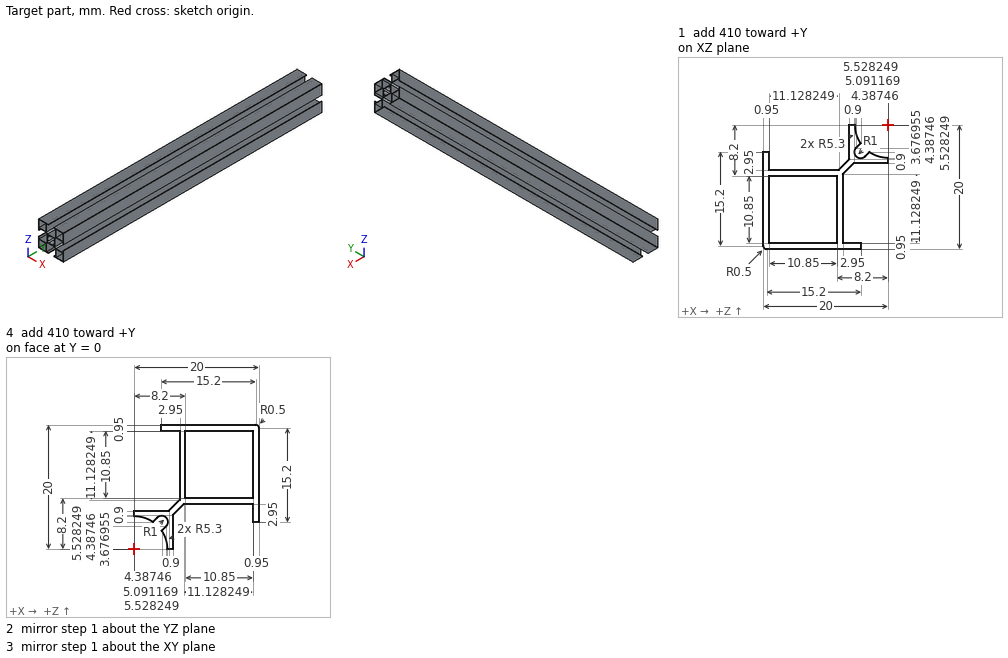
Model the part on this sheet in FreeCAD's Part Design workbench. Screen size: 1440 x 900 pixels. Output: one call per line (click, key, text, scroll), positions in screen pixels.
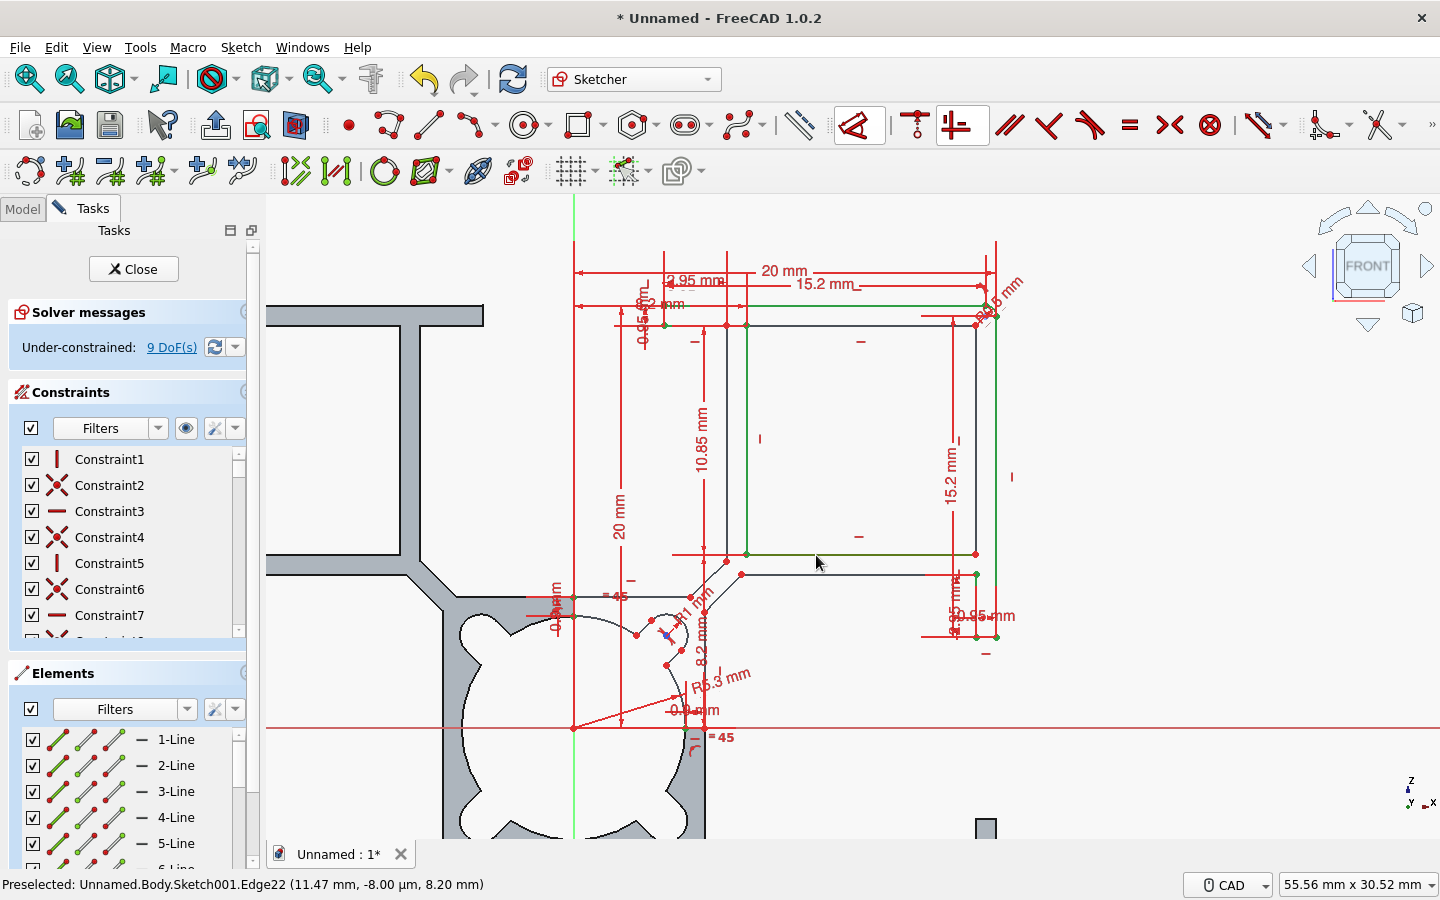
click(880, 126)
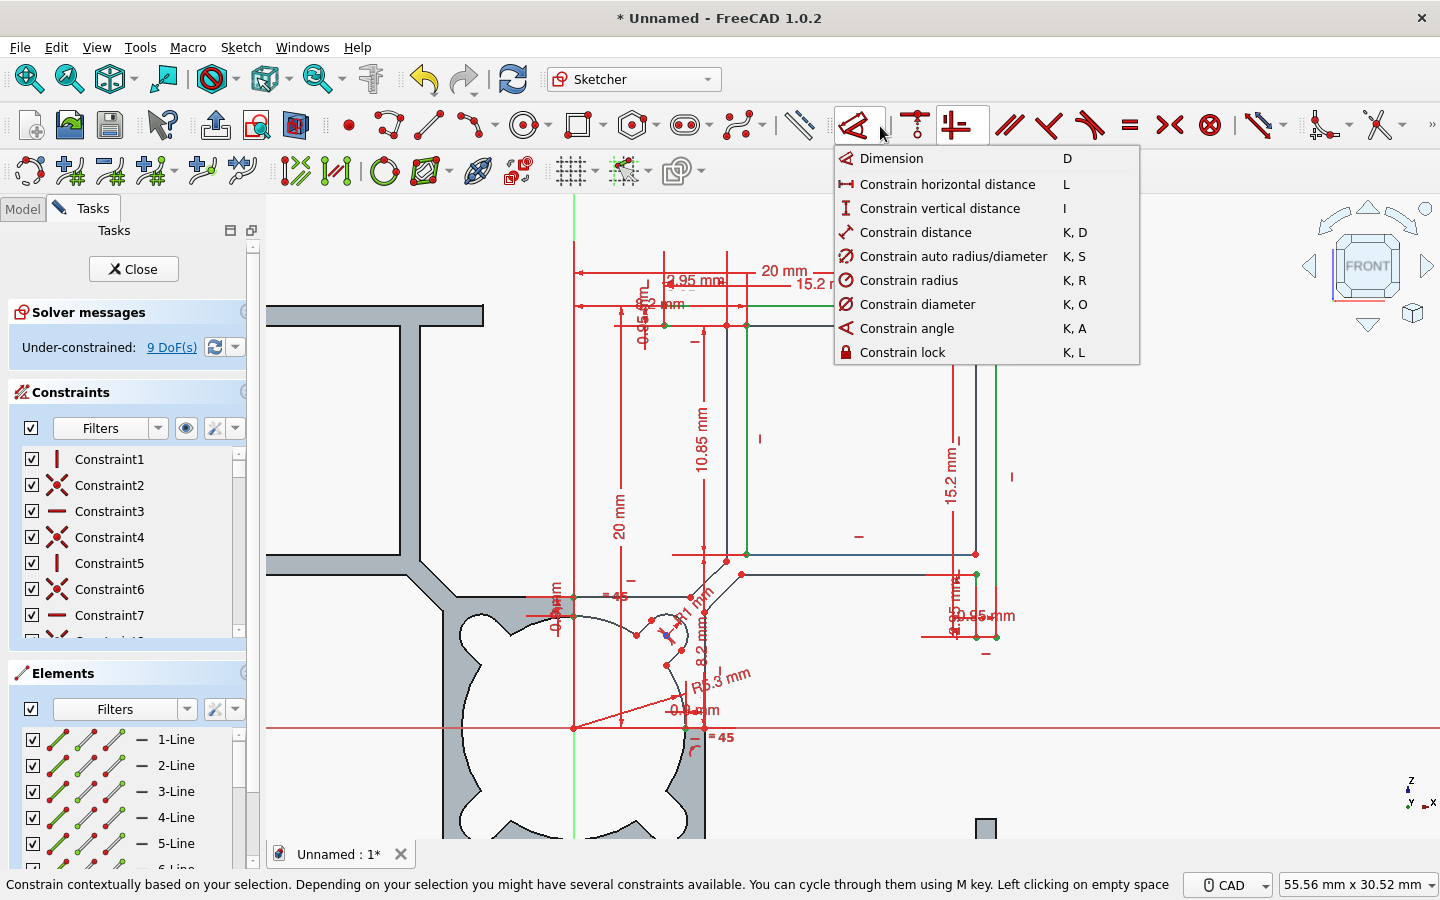
click(987, 184)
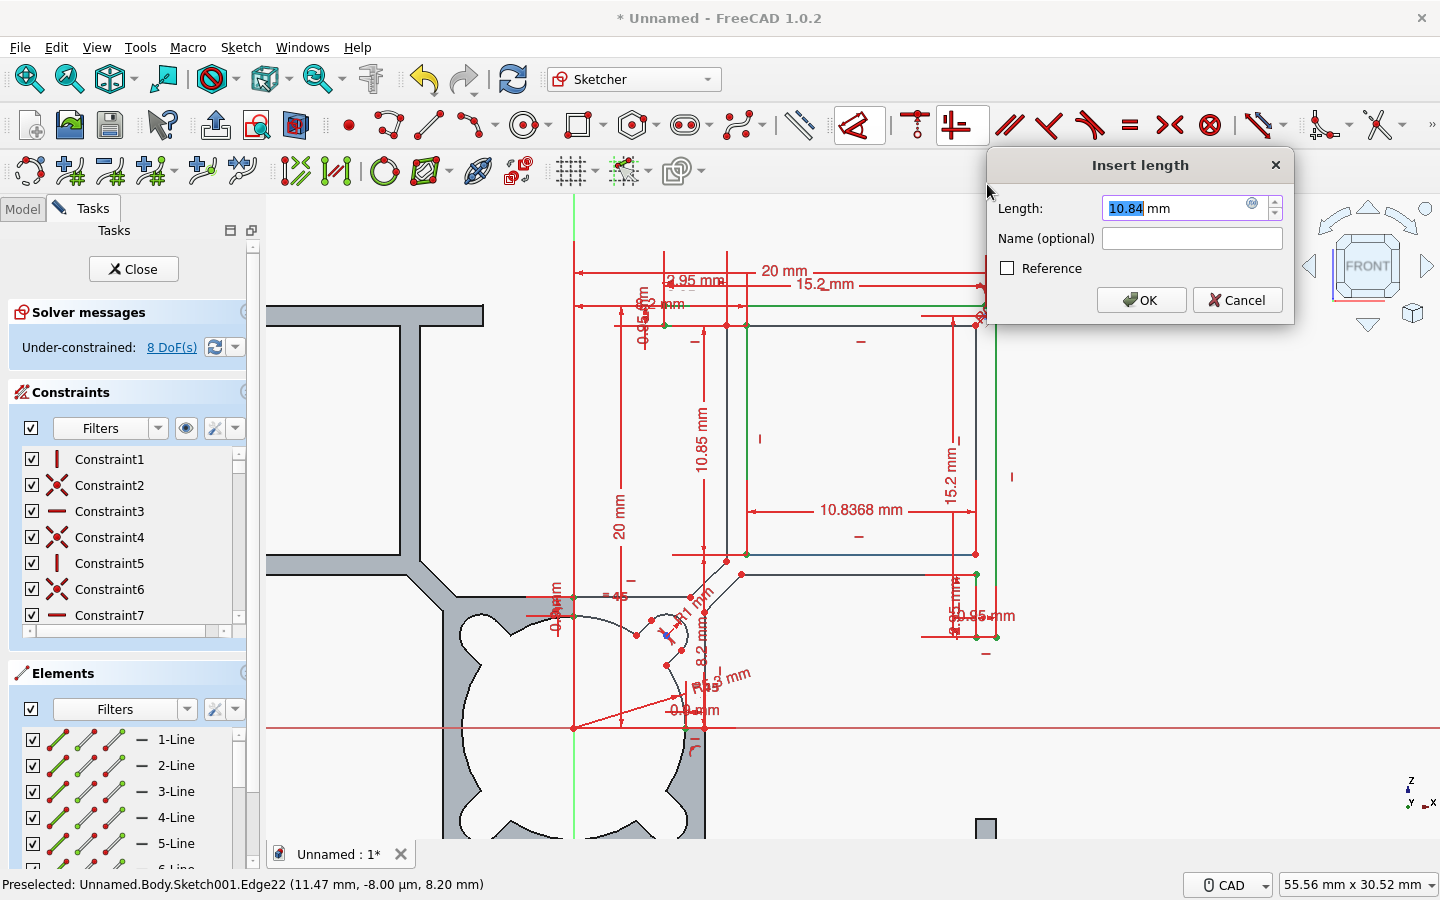
text(10.85)
key(Return)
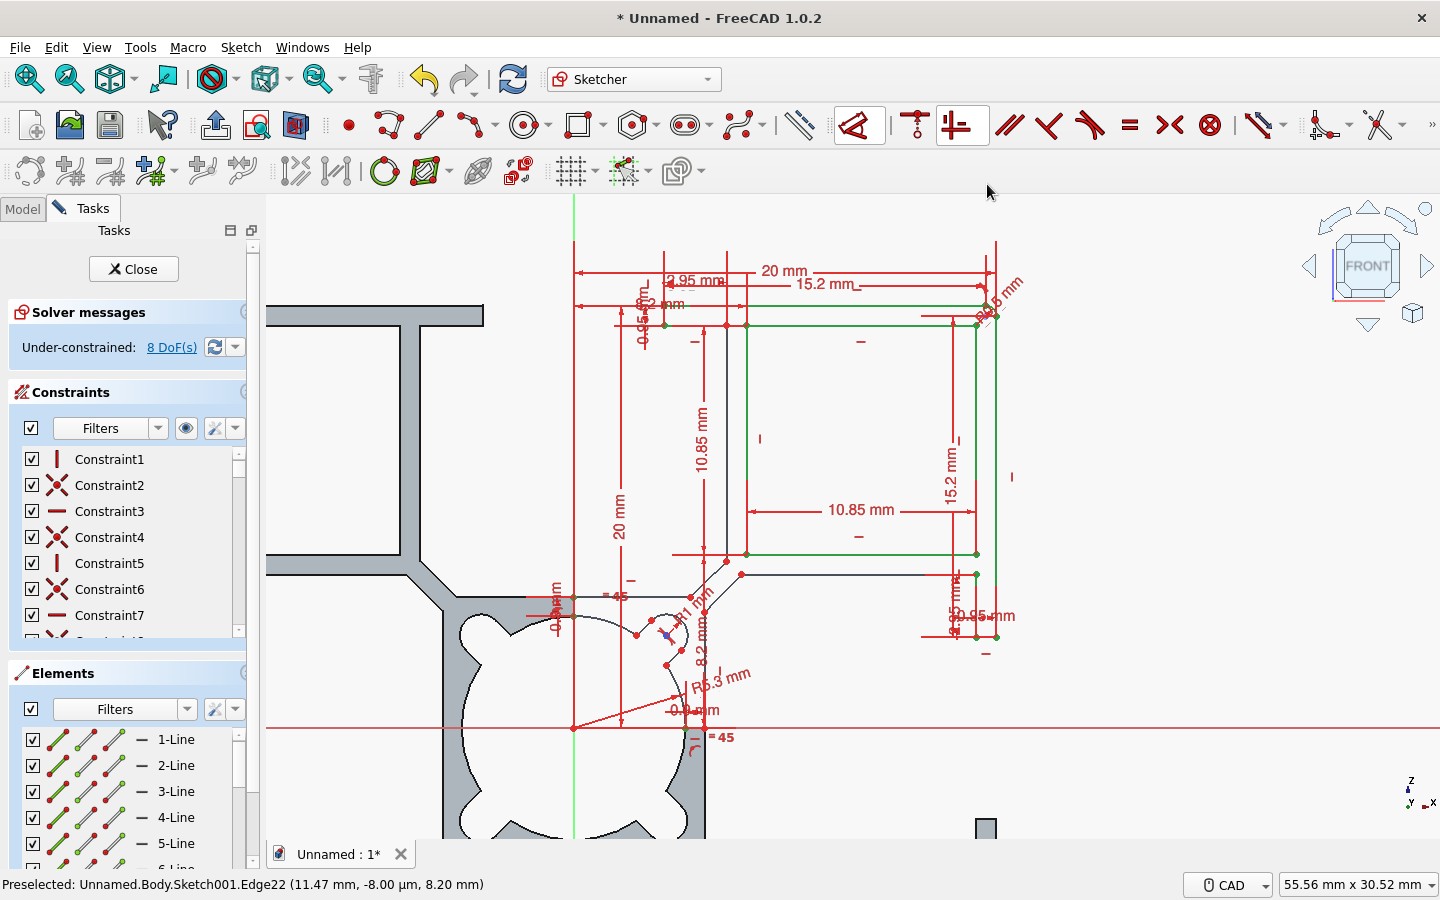
click(705, 670)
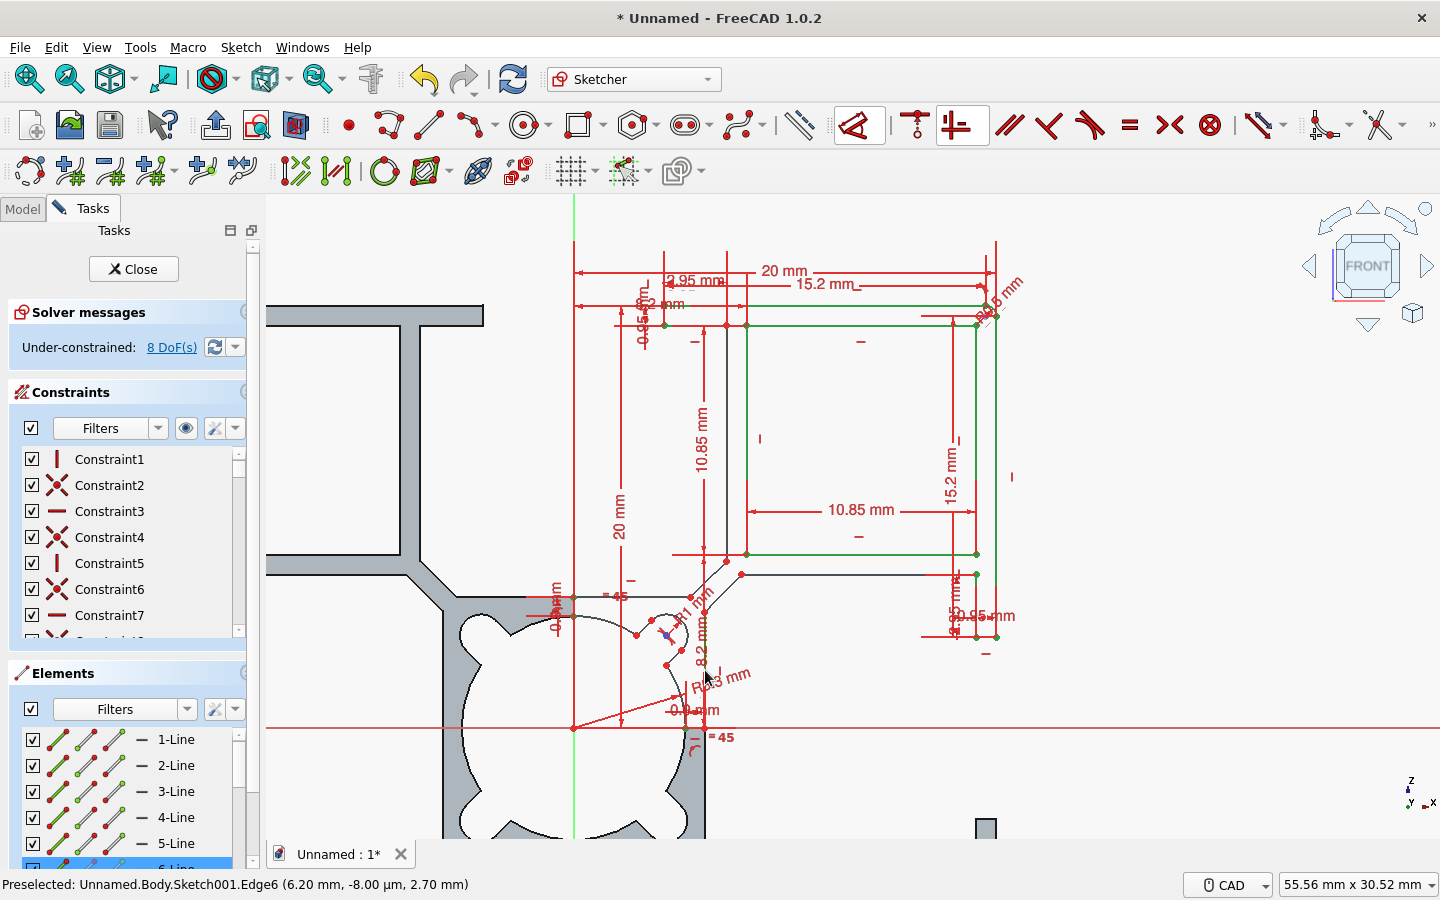
click(880, 126)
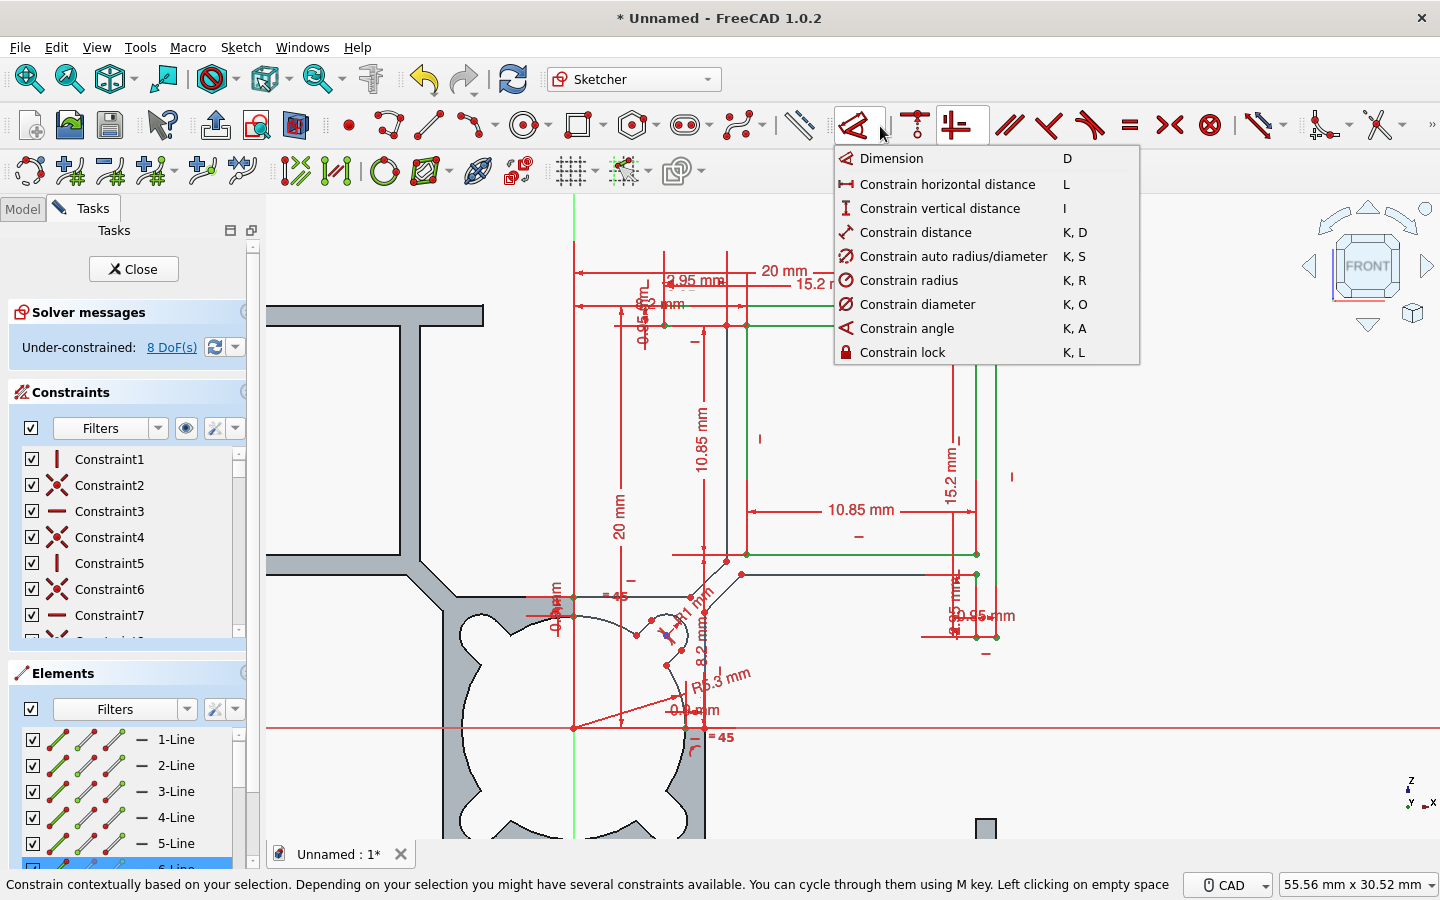
click(987, 208)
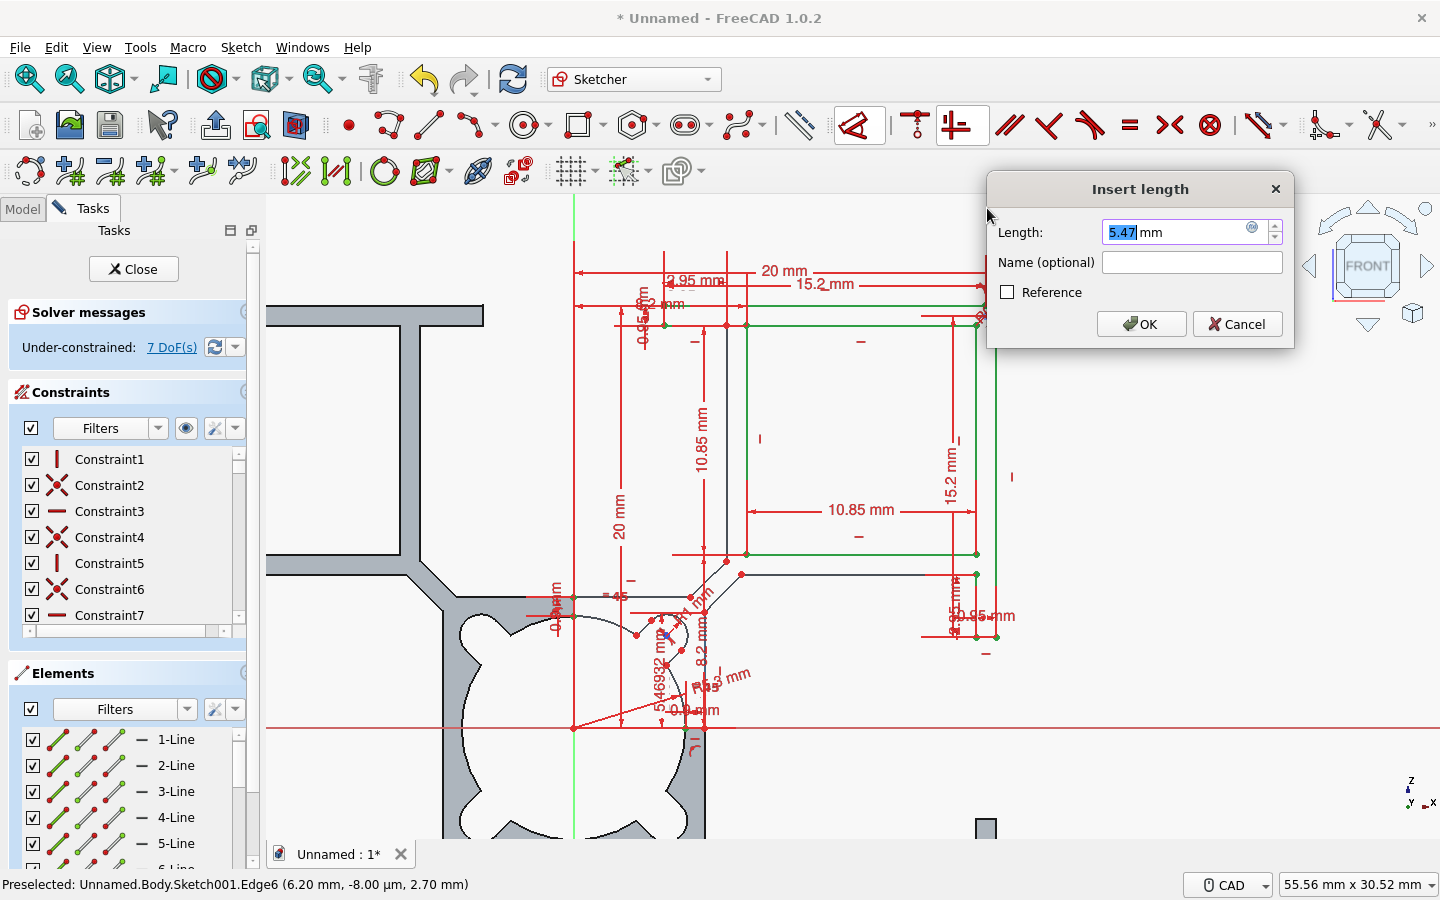
text(5.528249)
key(Return)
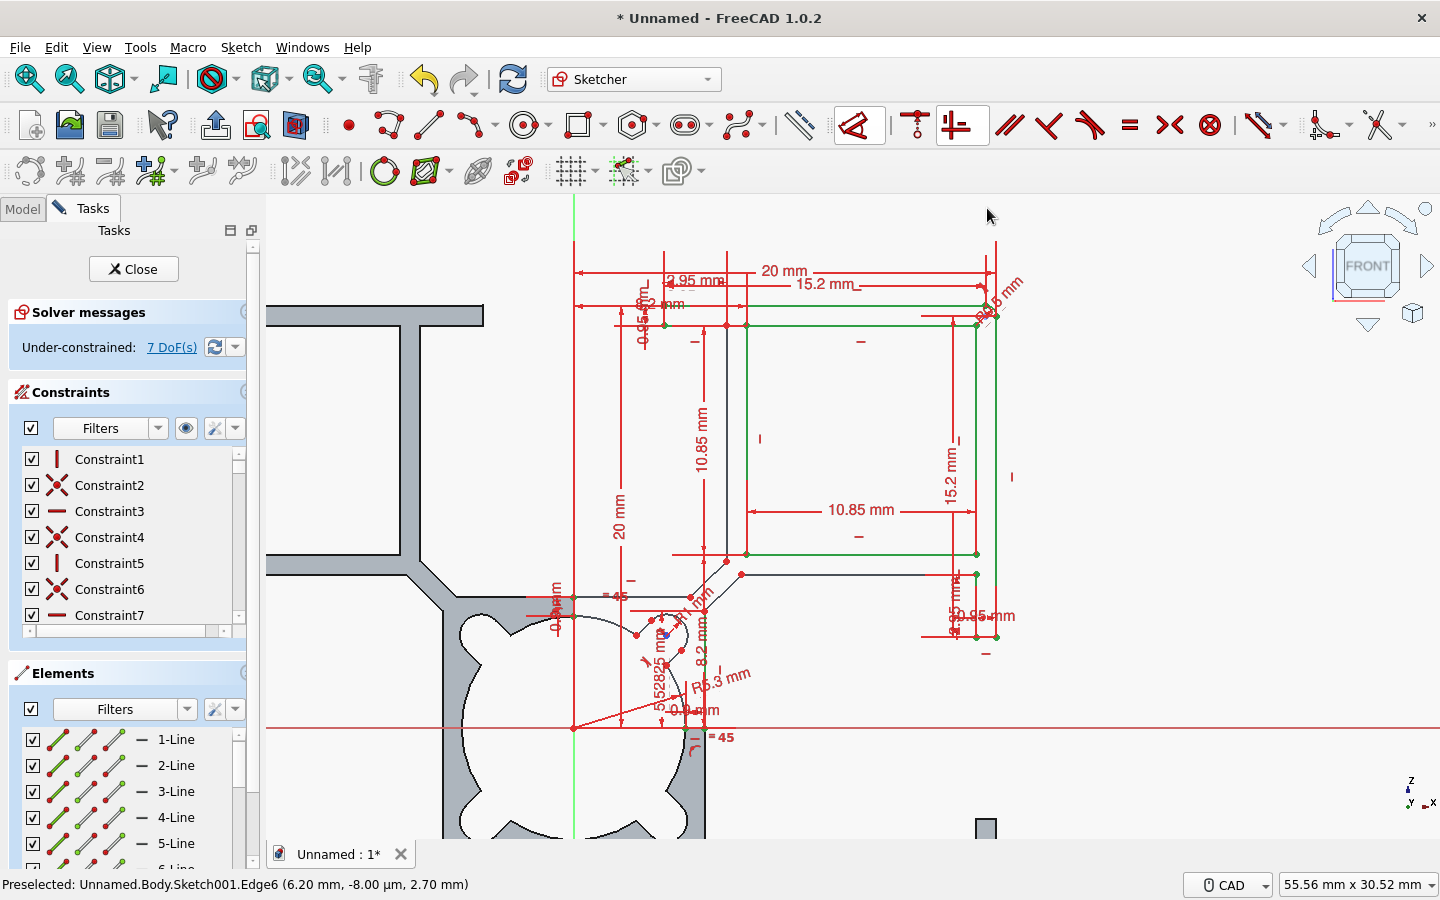
click(655, 597)